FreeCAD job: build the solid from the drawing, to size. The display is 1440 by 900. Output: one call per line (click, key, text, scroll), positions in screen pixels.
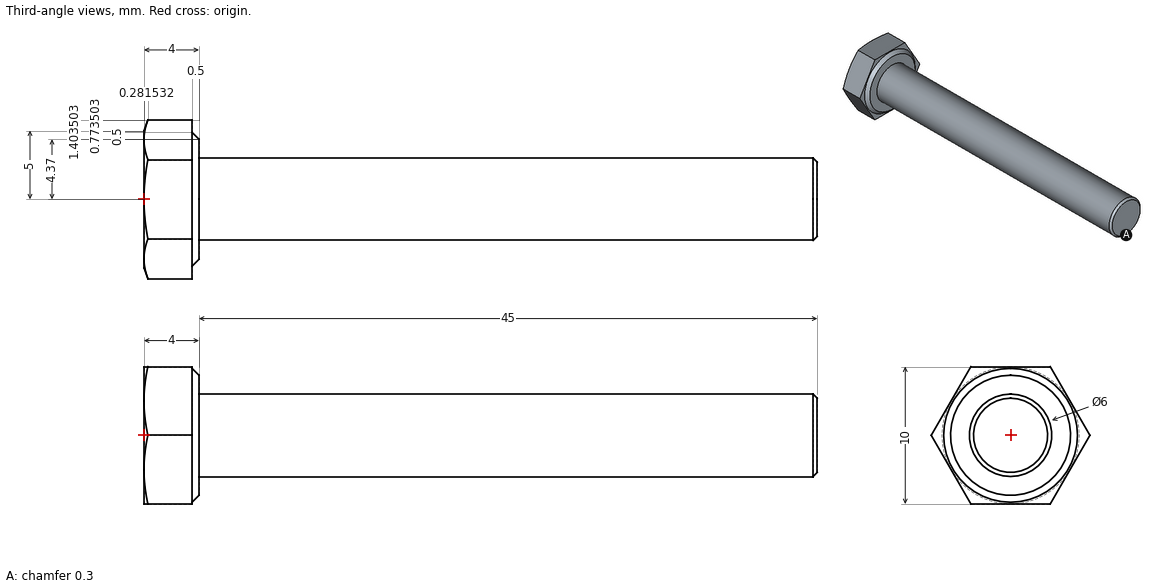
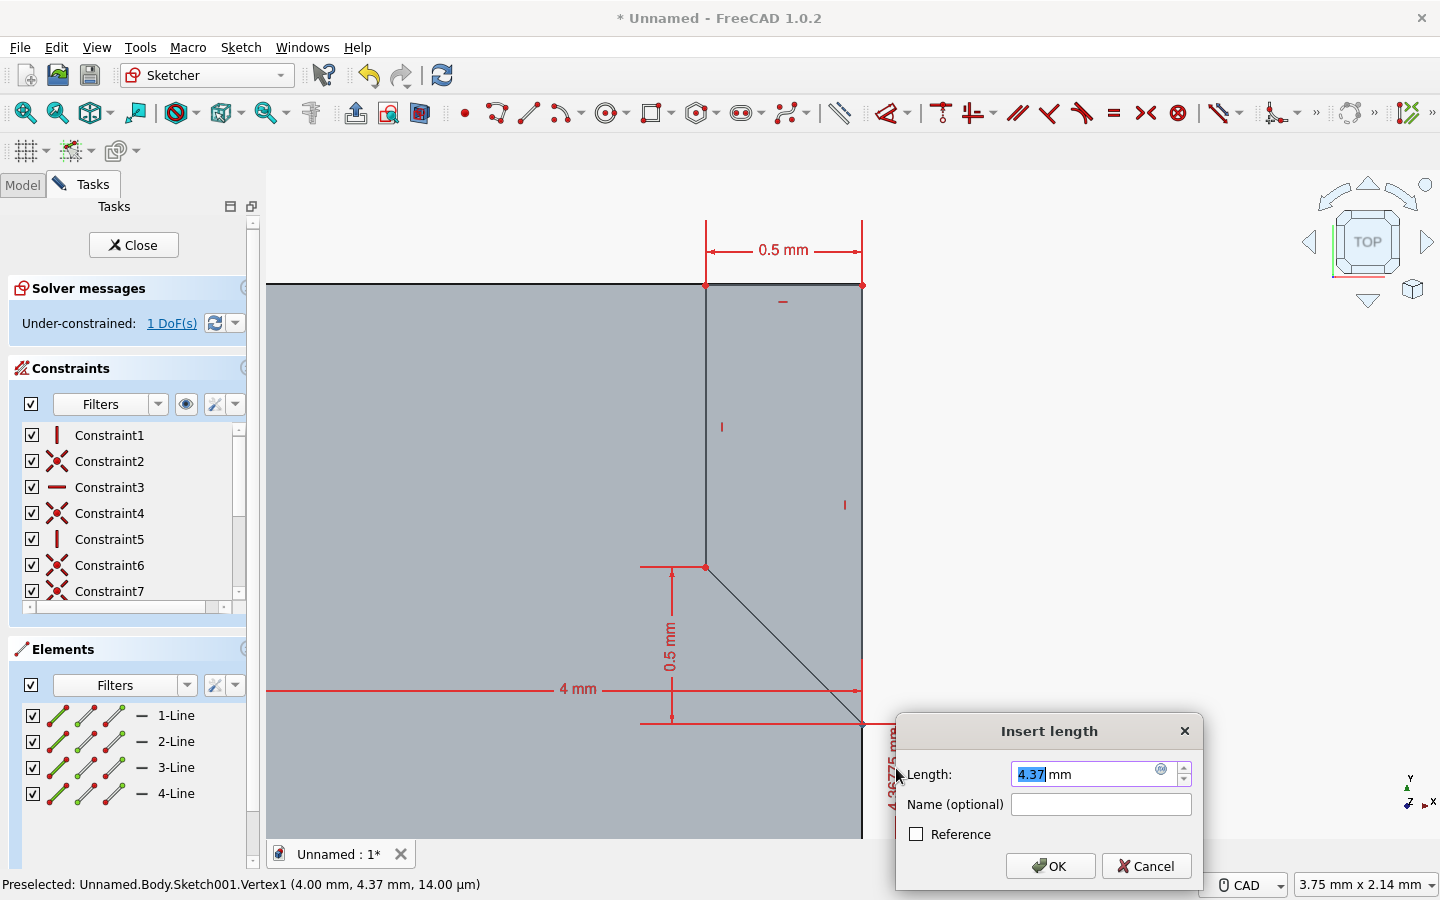
text(4.37)
key(Return)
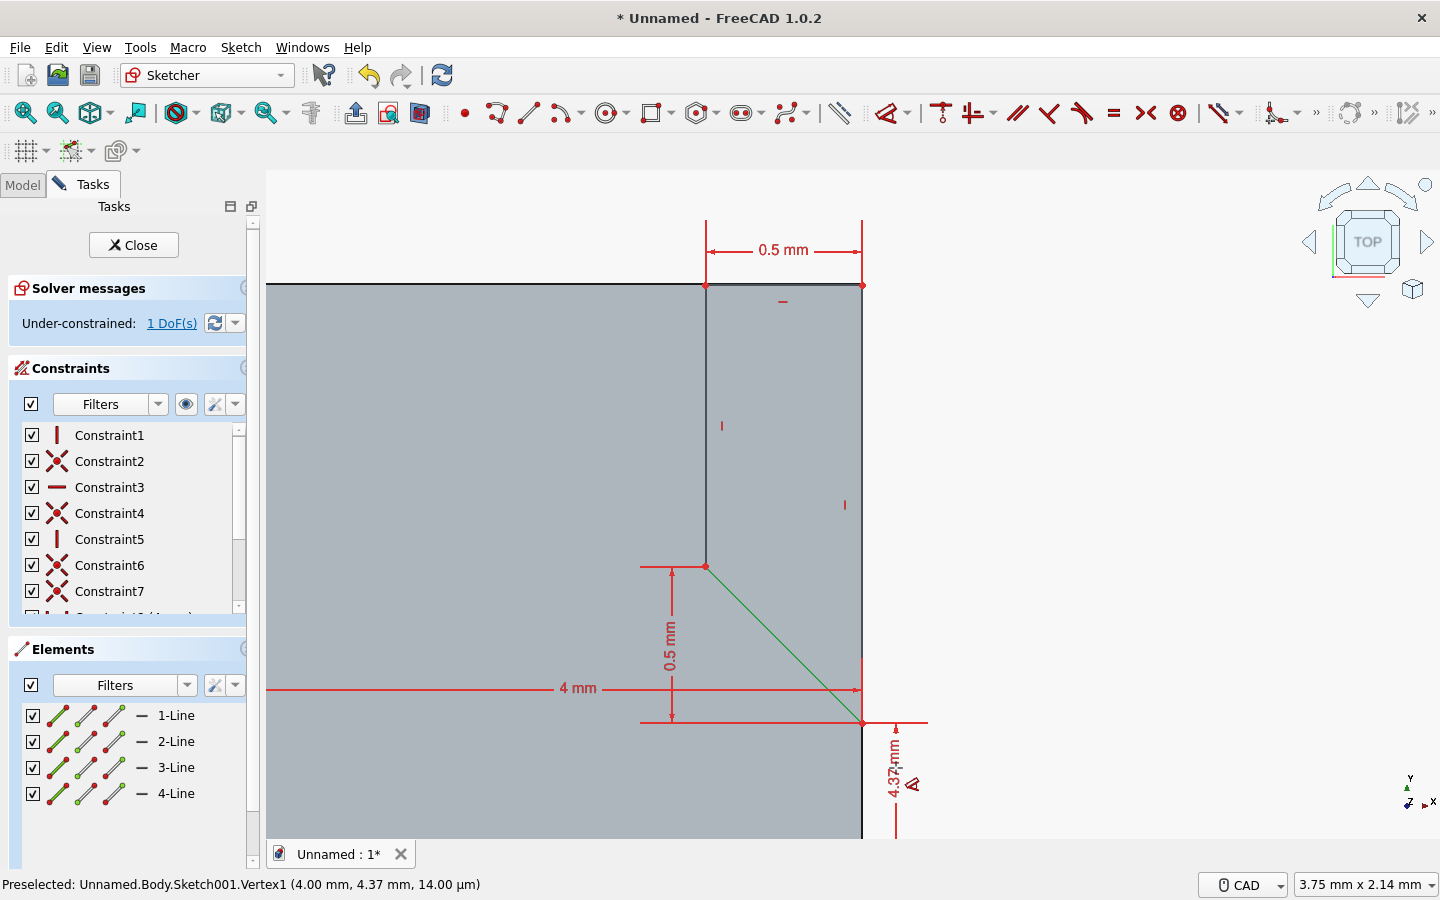
click(862, 592)
click(896, 504)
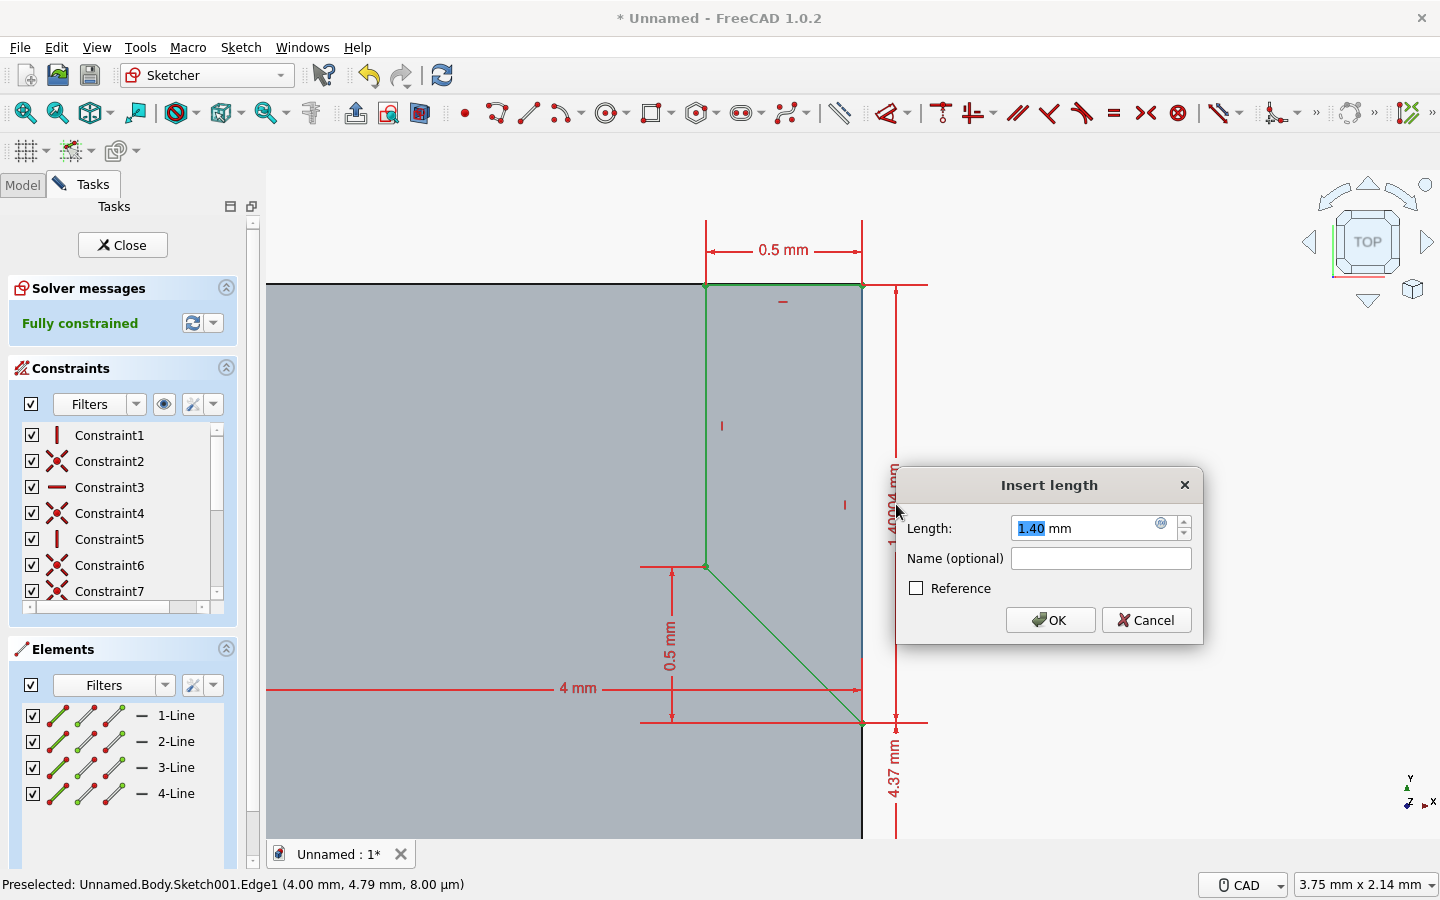
text(1.403503)
key(Return)
key(Escape)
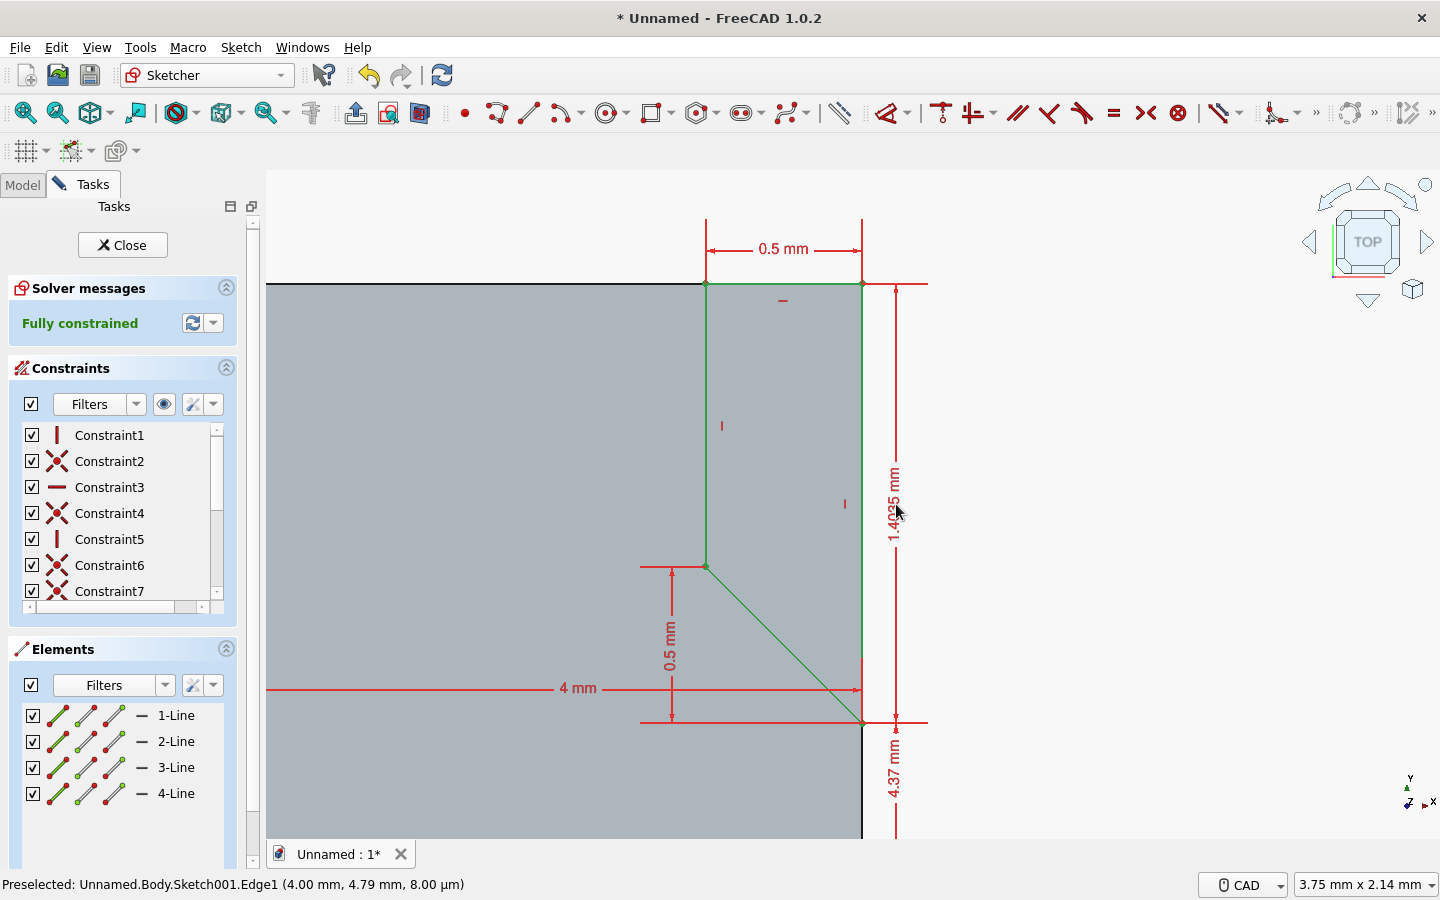
click(123, 245)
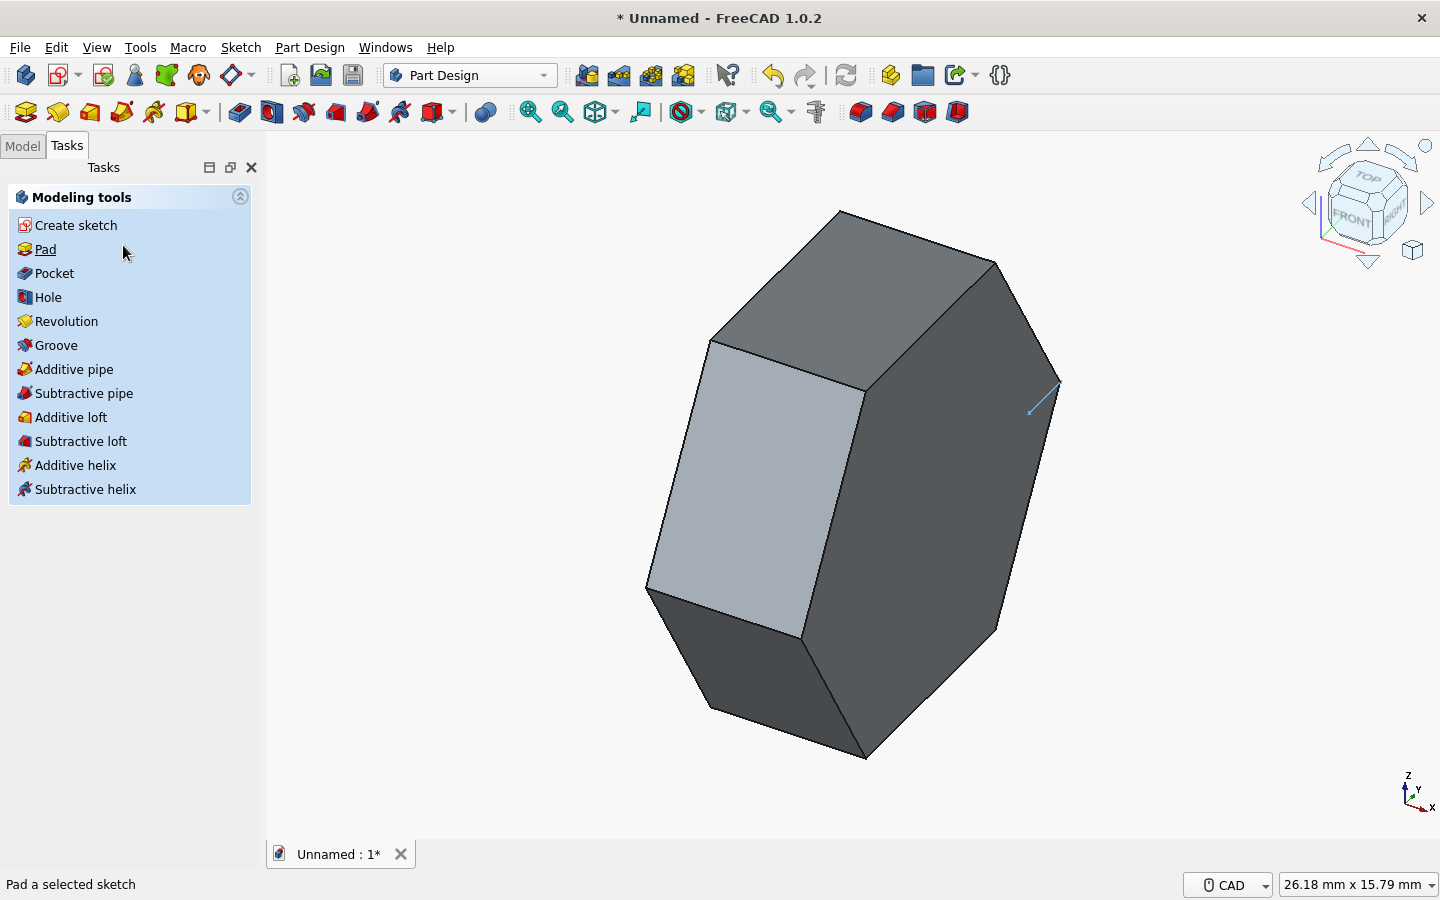
click(304, 112)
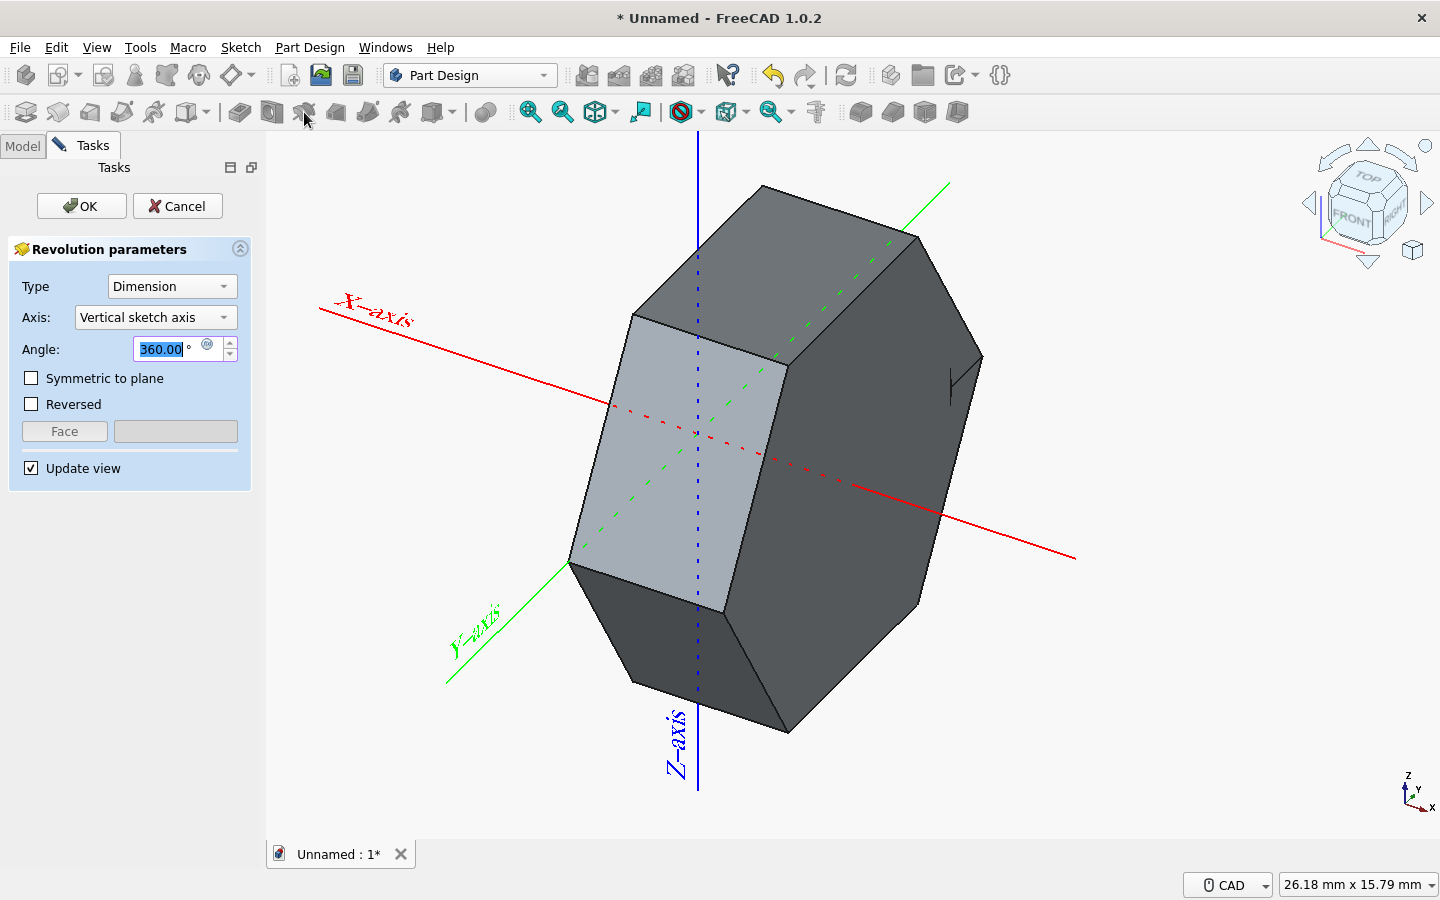
click(156, 318)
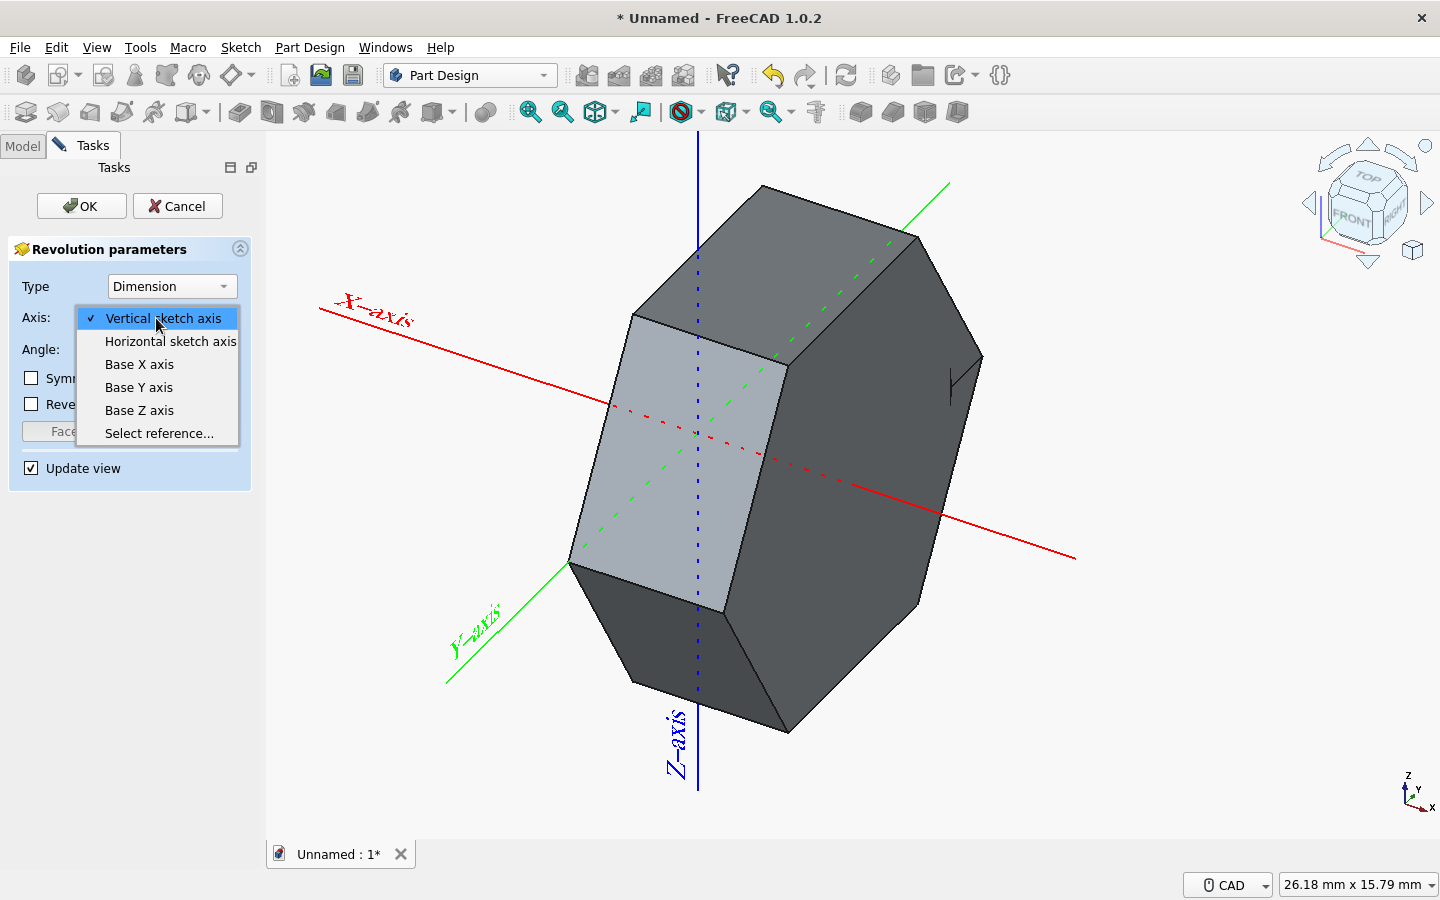
click(156, 342)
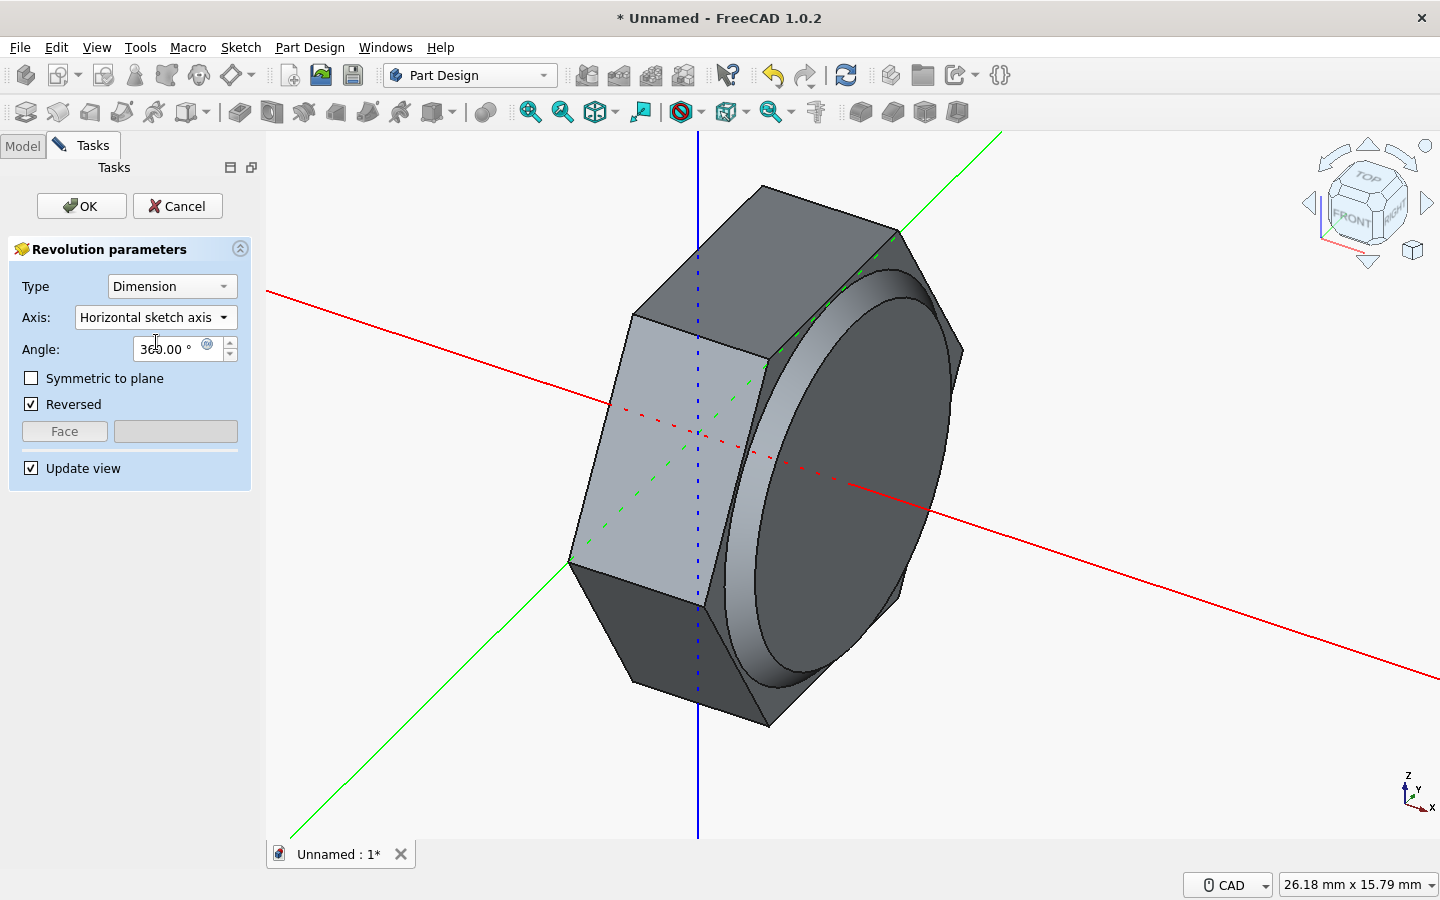
click(82, 206)